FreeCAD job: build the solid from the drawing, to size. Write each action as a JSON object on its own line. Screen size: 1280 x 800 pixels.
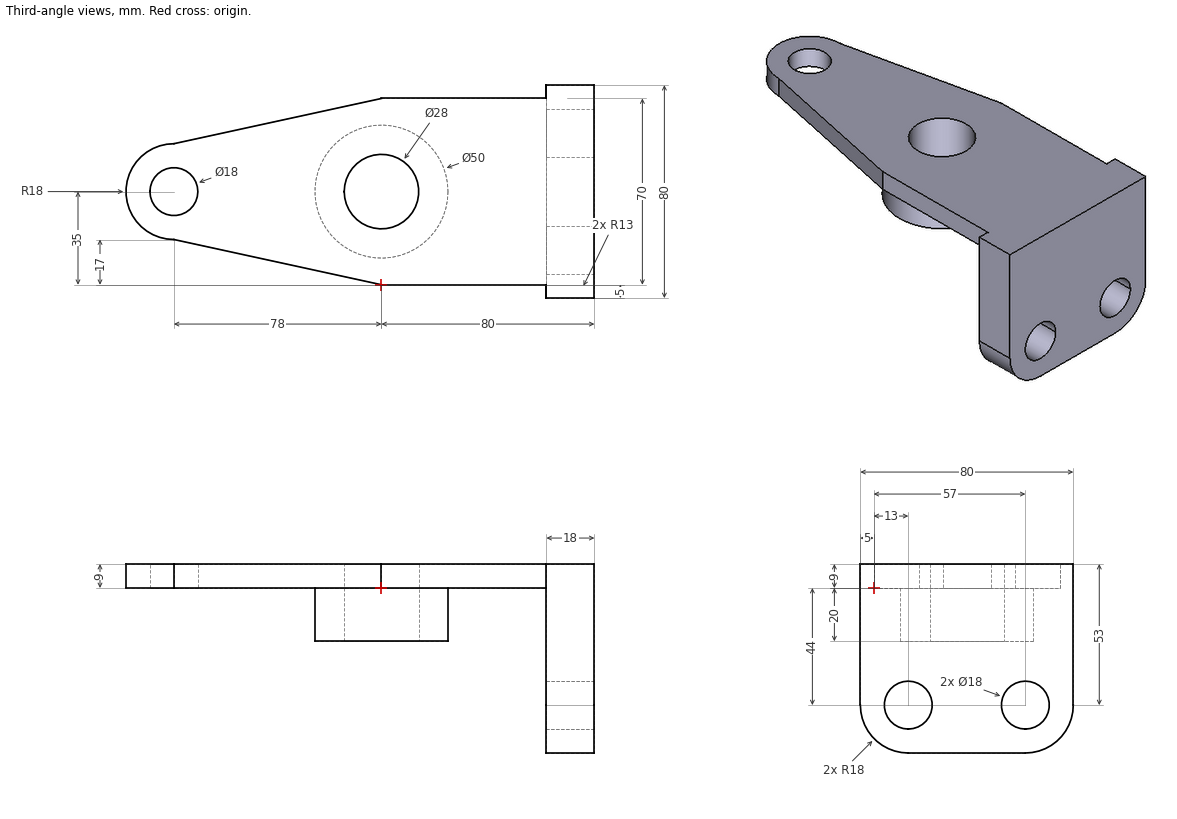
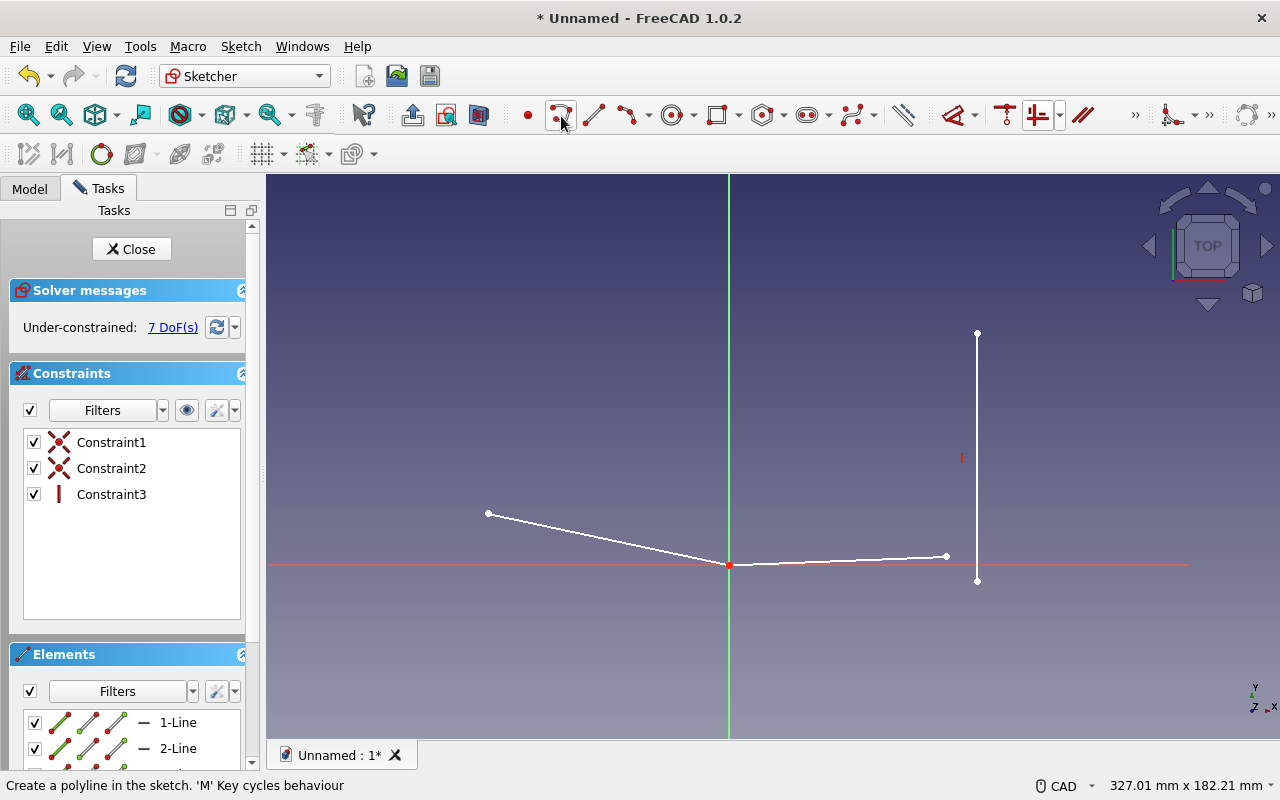
{"action": "left_click", "coordinate": [946, 348]}
{"action": "left_click", "coordinate": [729, 348]}
{"action": "left_click", "coordinate": [488, 401]}
{"action": "right_click", "coordinate": [488, 401]}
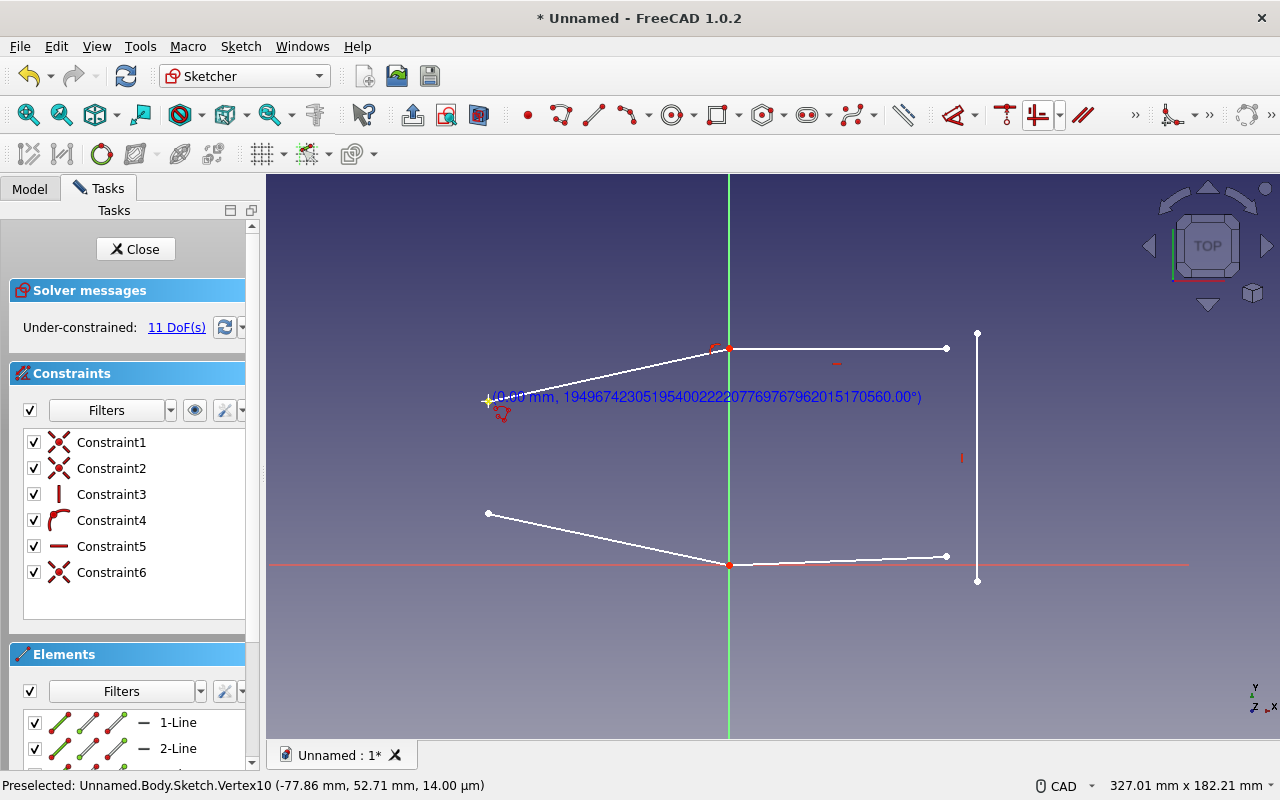
{"action": "left_click", "coordinate": [626, 116]}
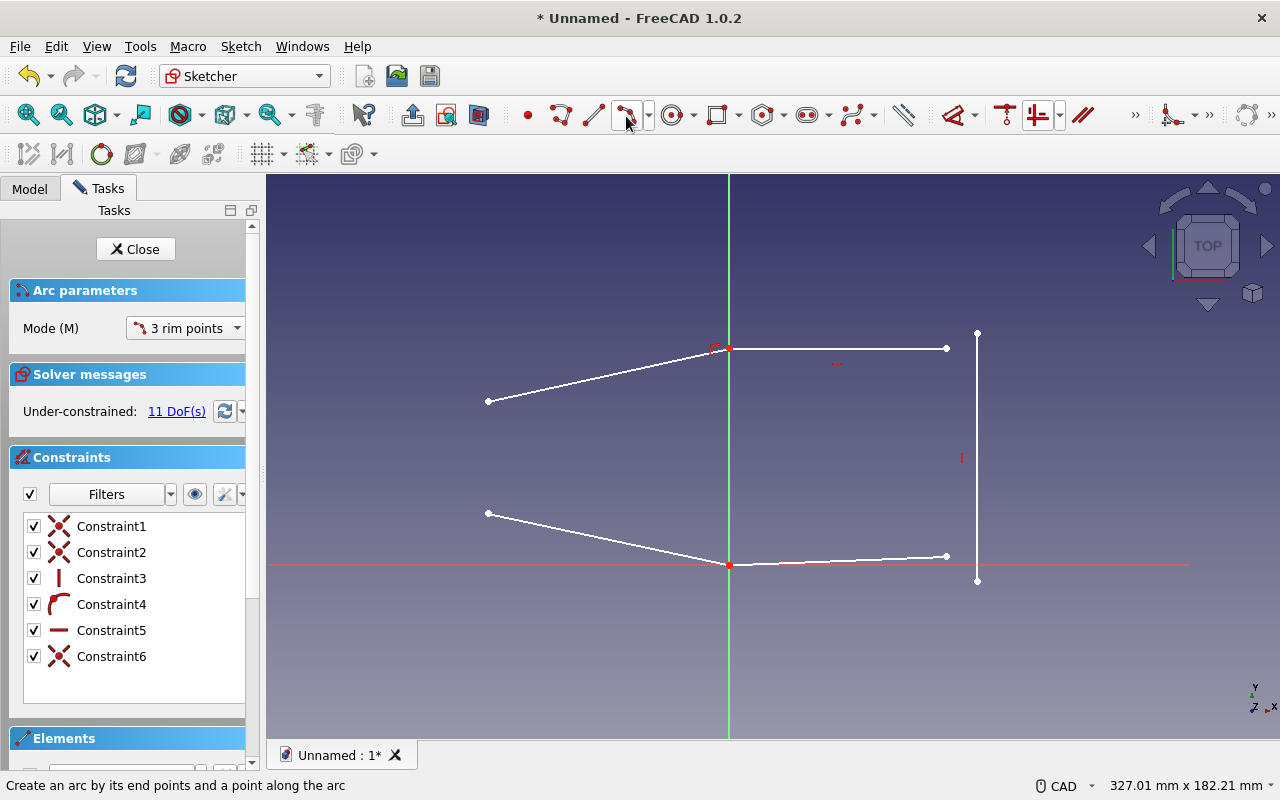
{"action": "left_click", "coordinate": [946, 557]}
{"action": "left_click", "coordinate": [977, 582]}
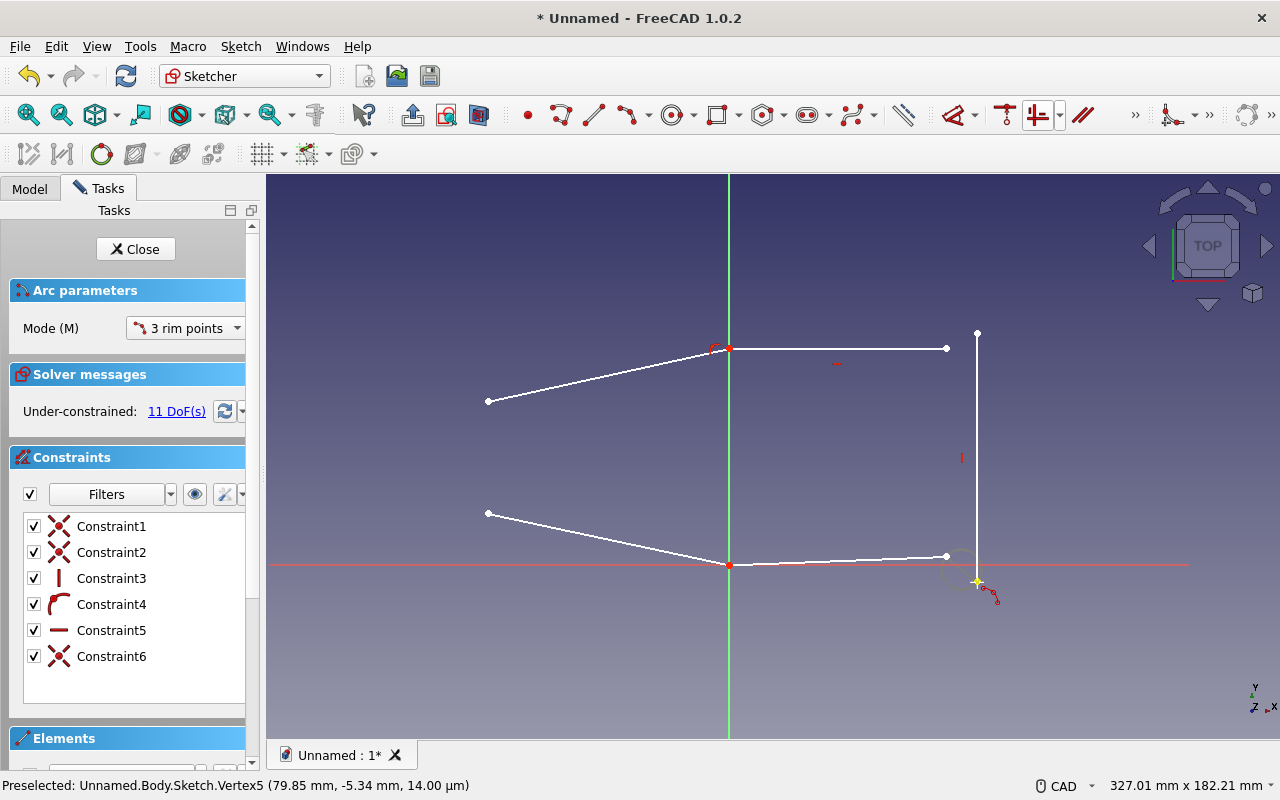
{"action": "scroll", "coordinate": [963, 570], "scroll_direction": "up", "scroll_amount": 7}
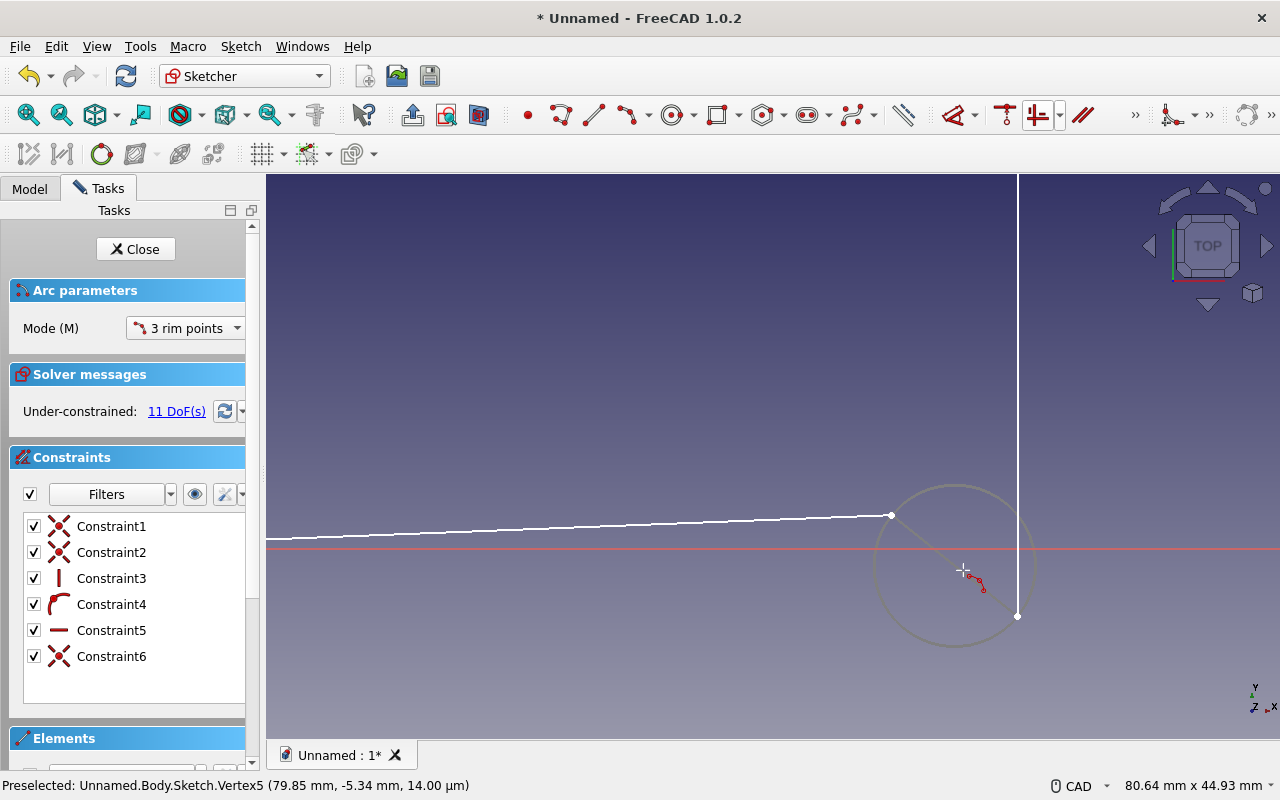
{"action": "left_click", "coordinate": [962, 566]}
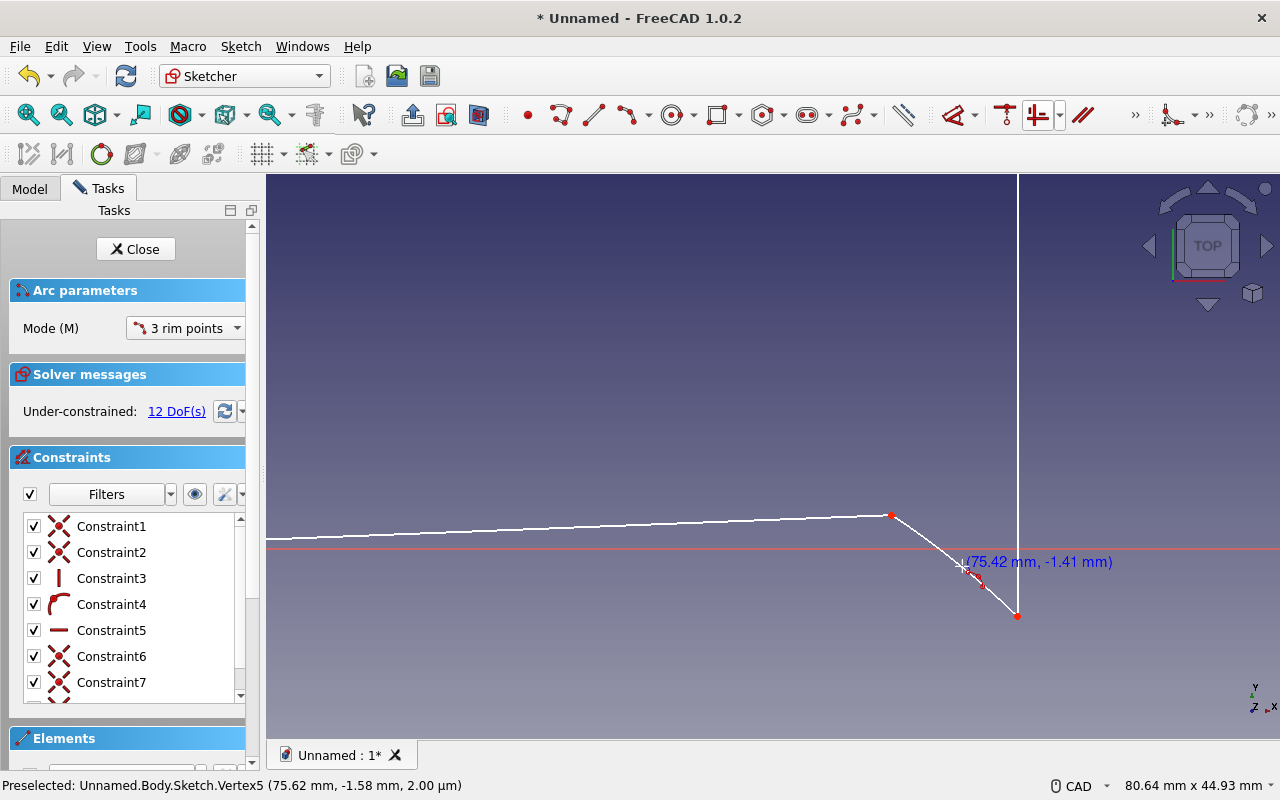
{"action": "scroll", "coordinate": [964, 570], "scroll_direction": "down", "scroll_amount": 7}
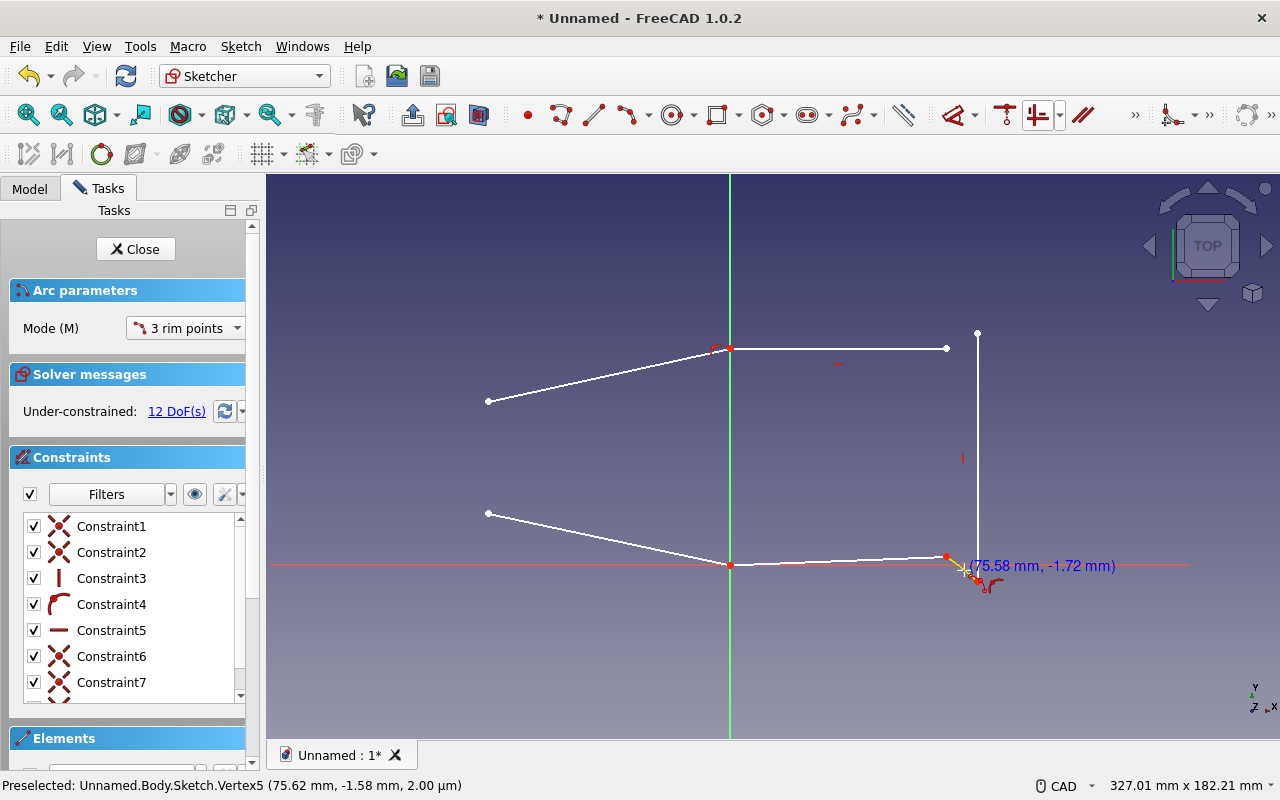
{"action": "left_click", "coordinate": [978, 334]}
{"action": "left_click", "coordinate": [947, 349]}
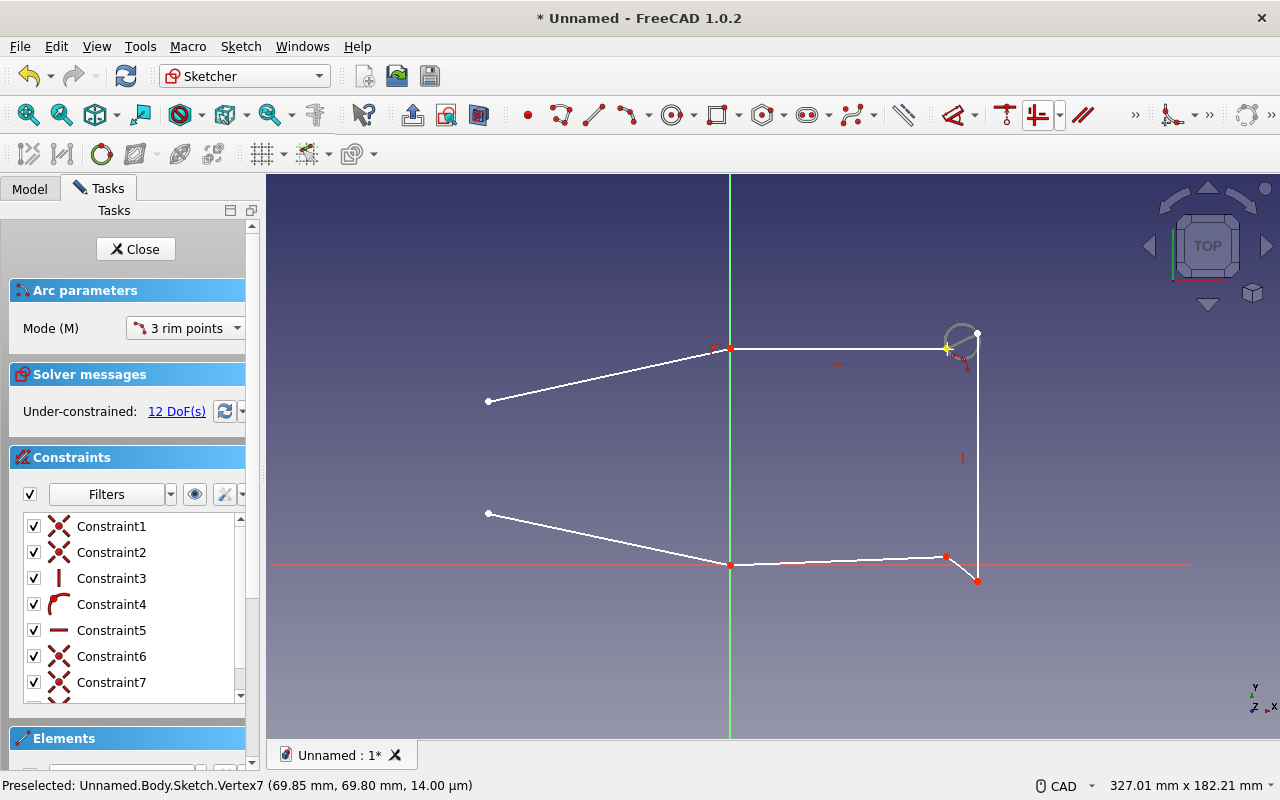
{"action": "scroll", "coordinate": [964, 344], "scroll_direction": "up", "scroll_amount": 7}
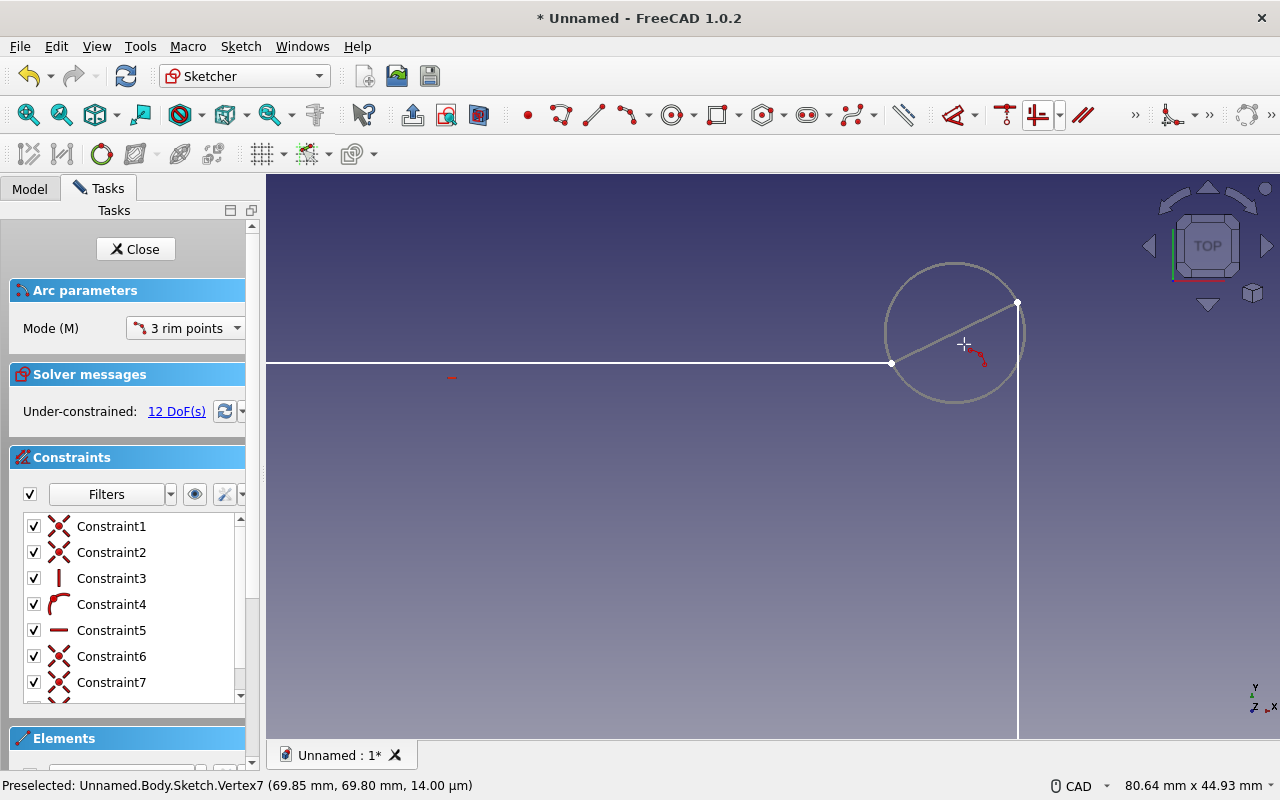
{"action": "left_click", "coordinate": [962, 344]}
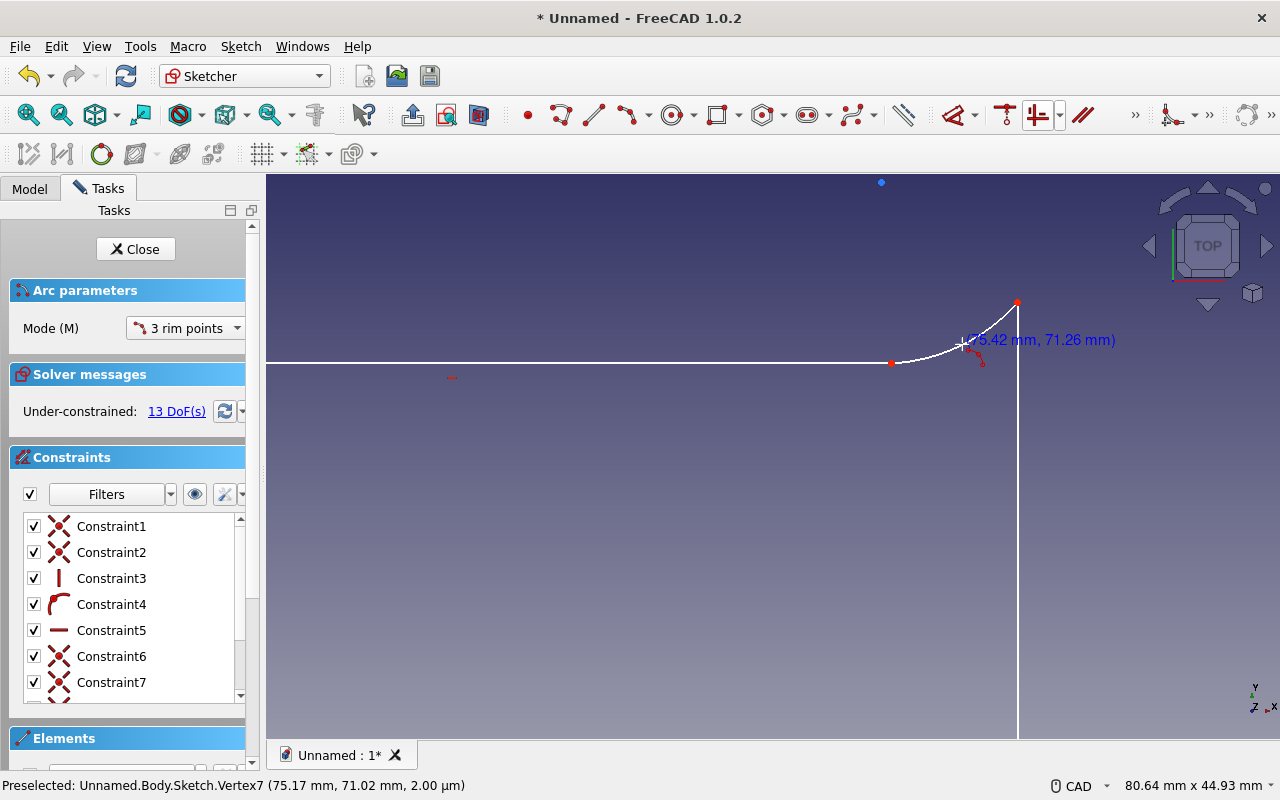
{"action": "scroll", "coordinate": [964, 344], "scroll_direction": "down", "scroll_amount": 7}